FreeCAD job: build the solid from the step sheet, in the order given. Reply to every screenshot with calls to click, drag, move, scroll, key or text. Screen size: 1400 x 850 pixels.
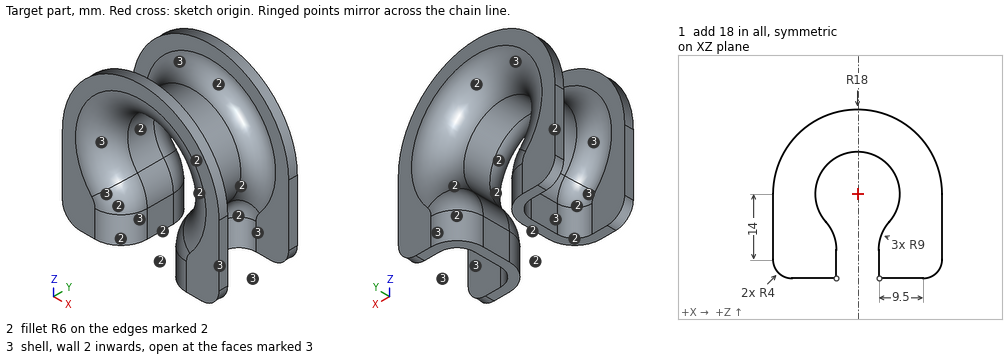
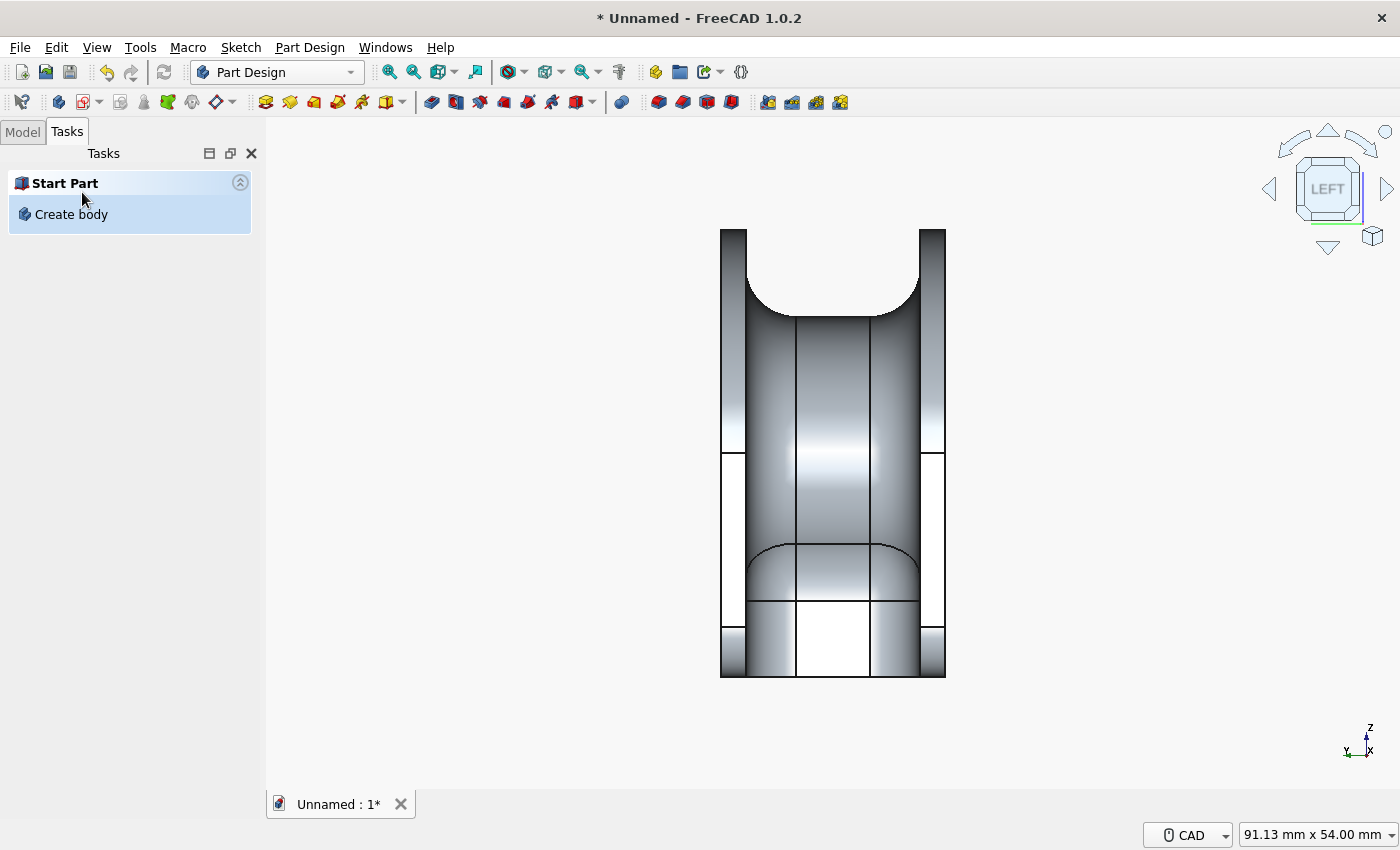
key(0)